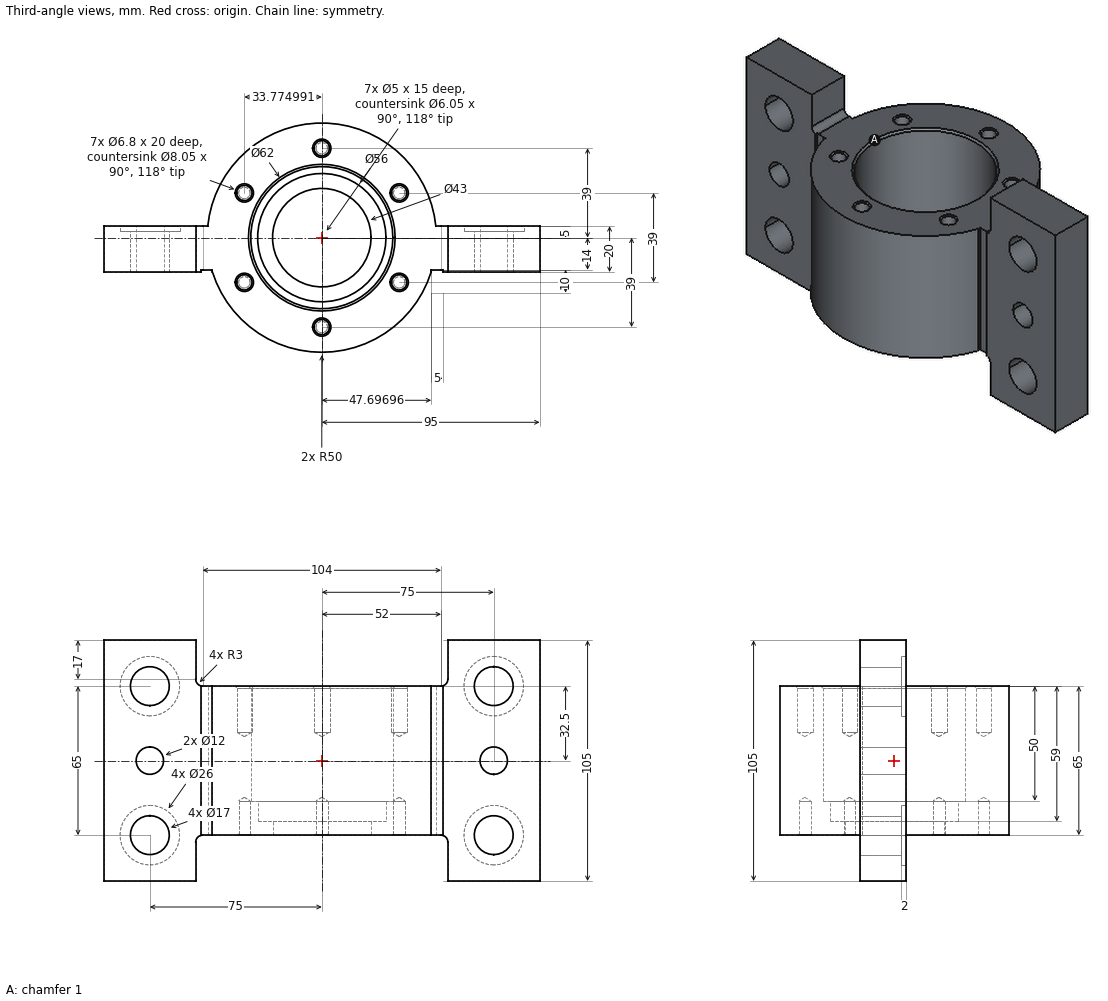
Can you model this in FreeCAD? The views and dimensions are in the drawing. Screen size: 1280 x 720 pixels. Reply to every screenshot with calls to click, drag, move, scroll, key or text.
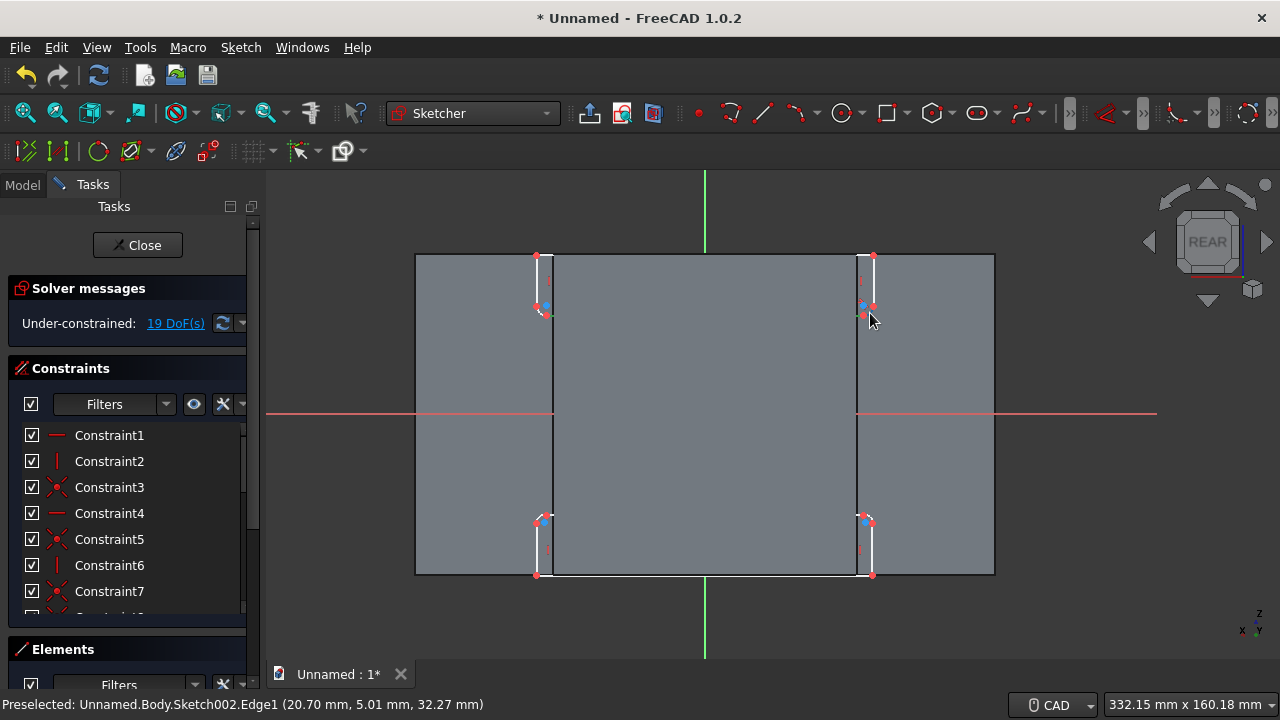
scroll(538, 311, up, 6)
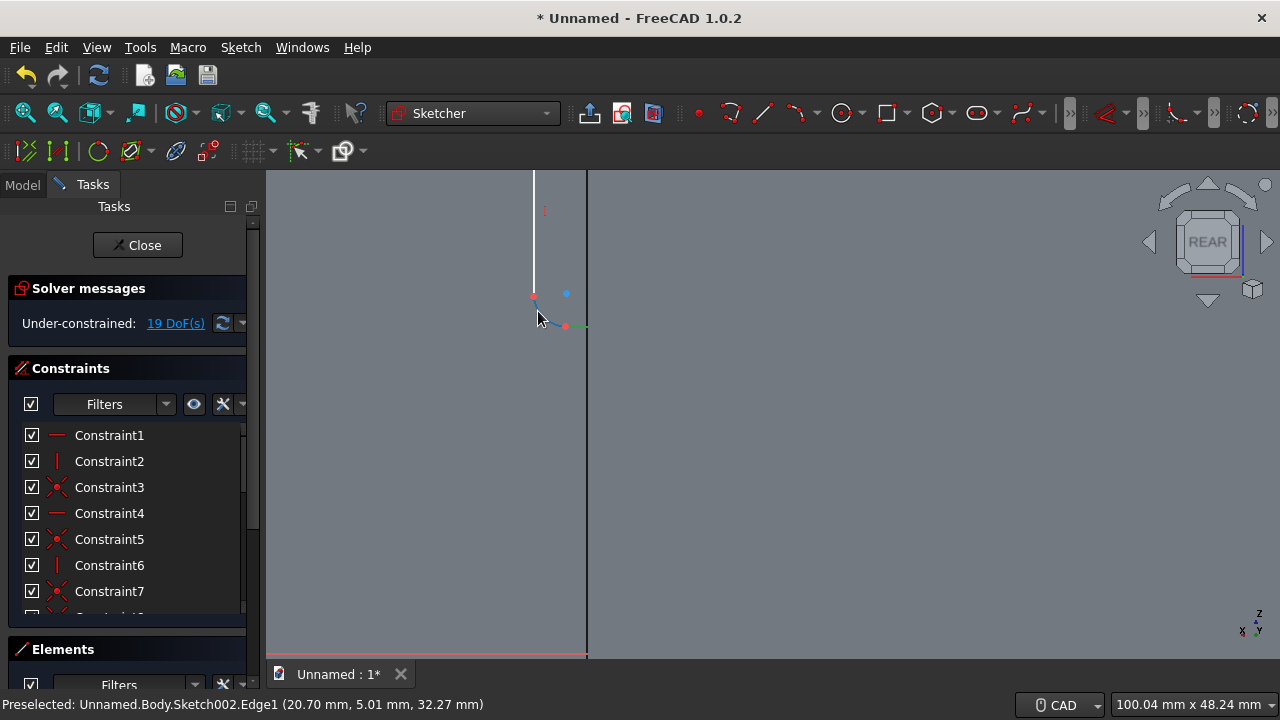
click(538, 310)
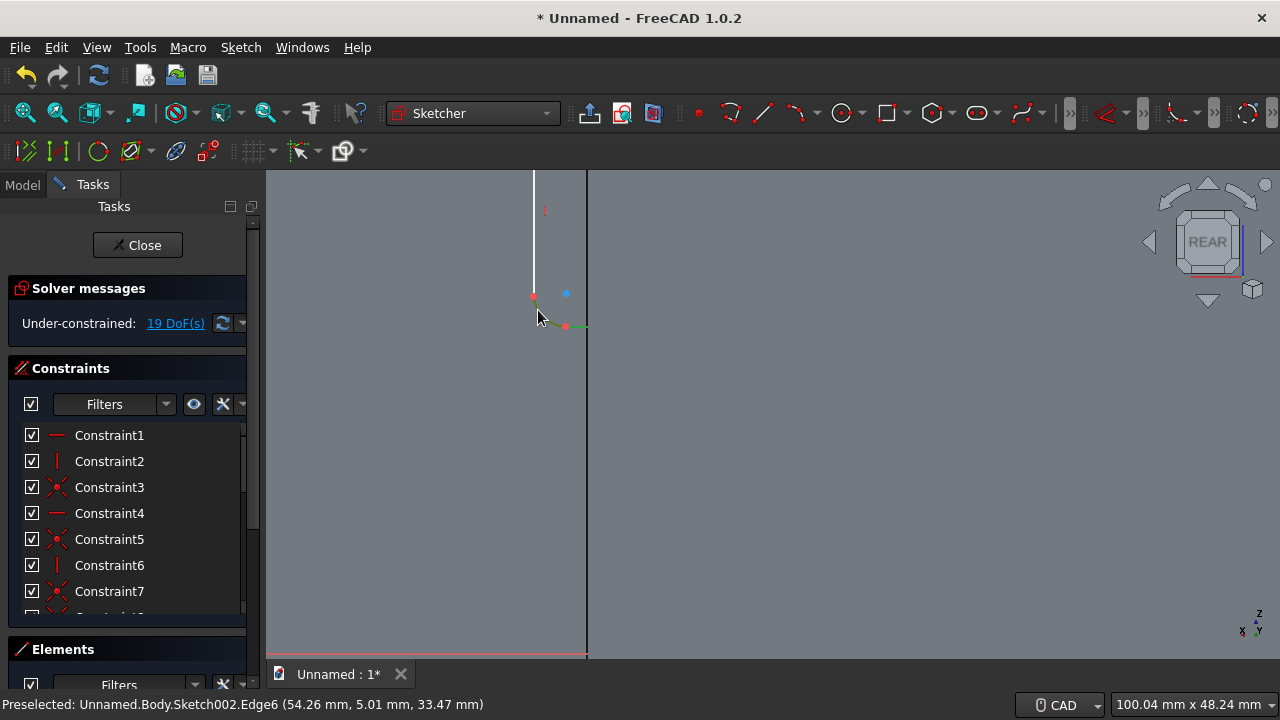
key(t)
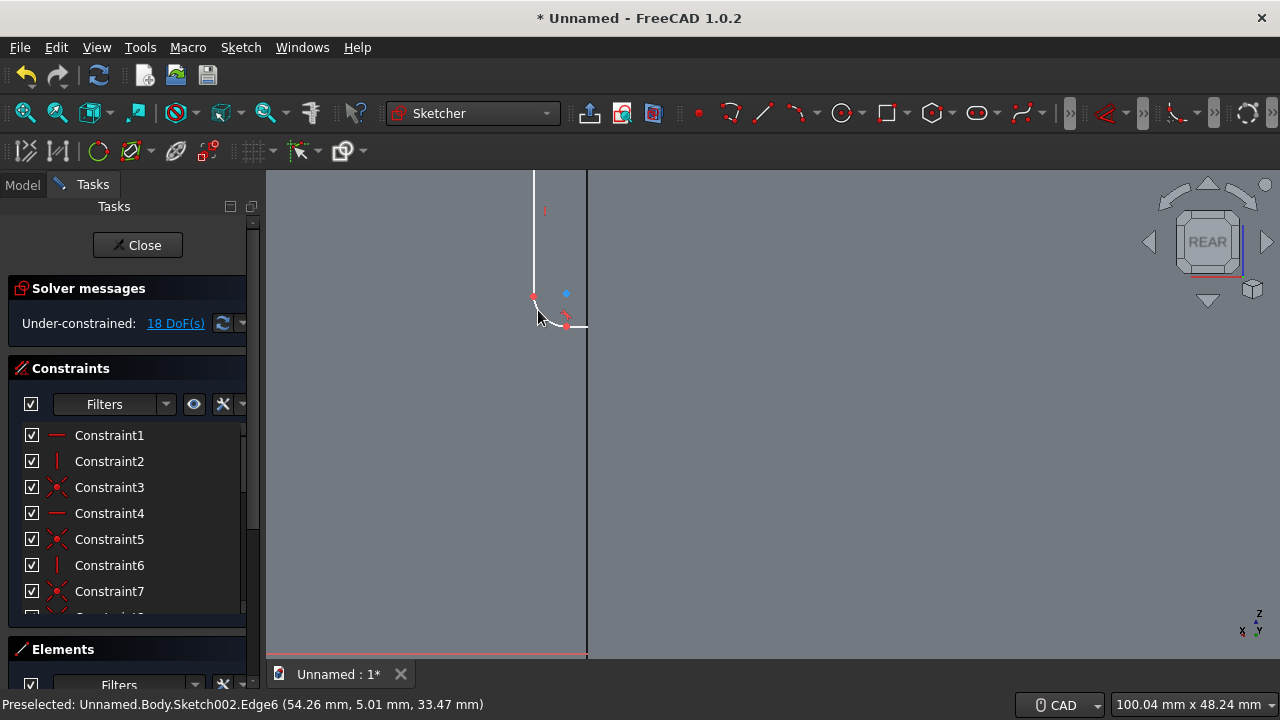
scroll(538, 311, down, 6)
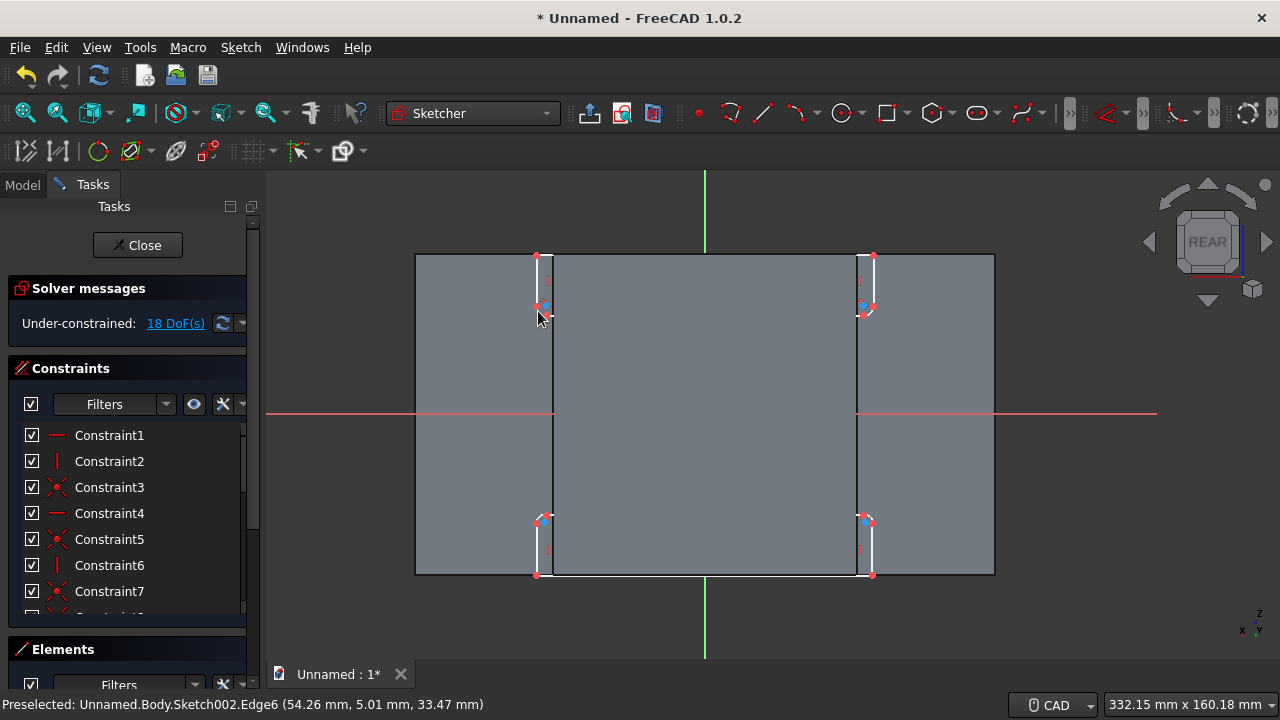
click(874, 291)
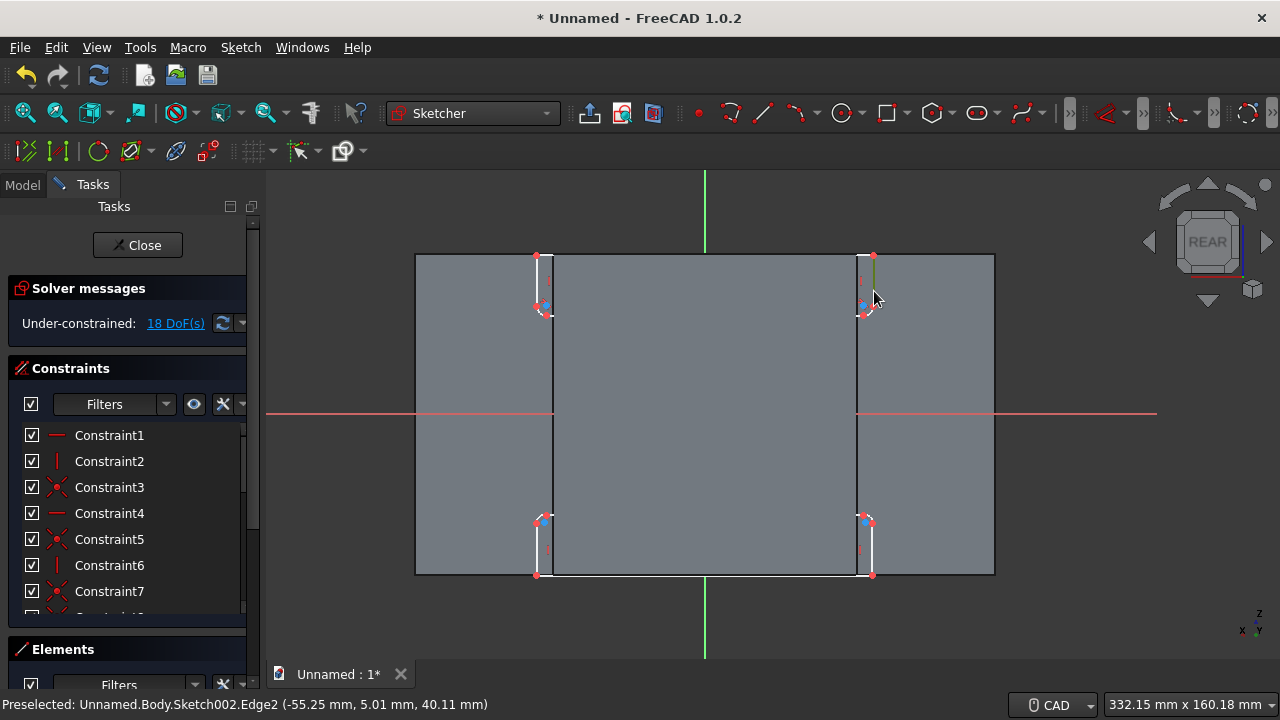
scroll(870, 313, up, 4)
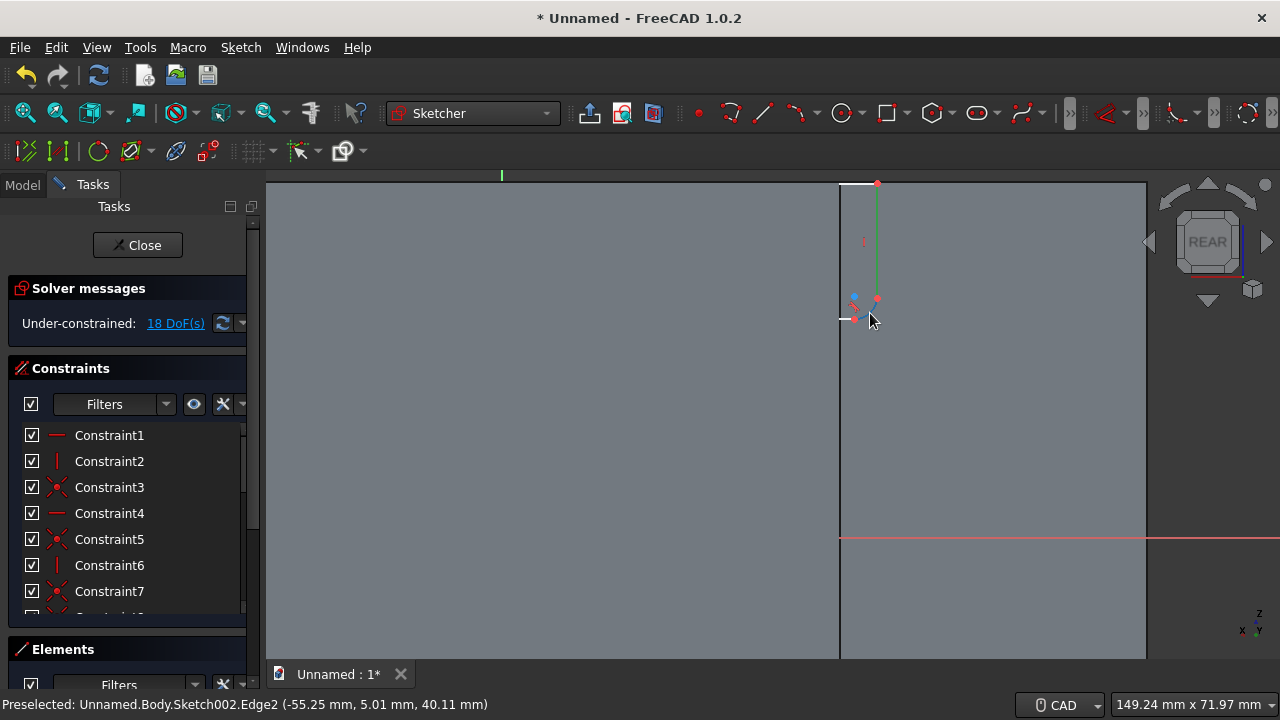
click(870, 313)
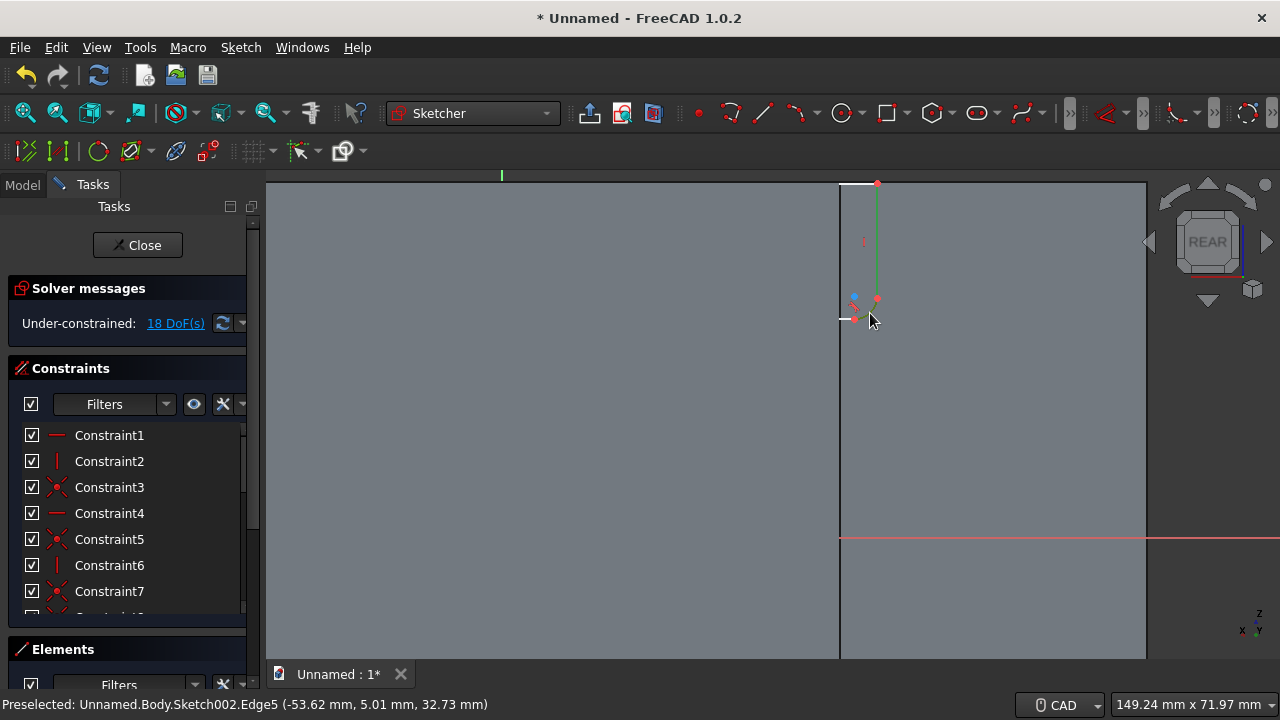
key(t)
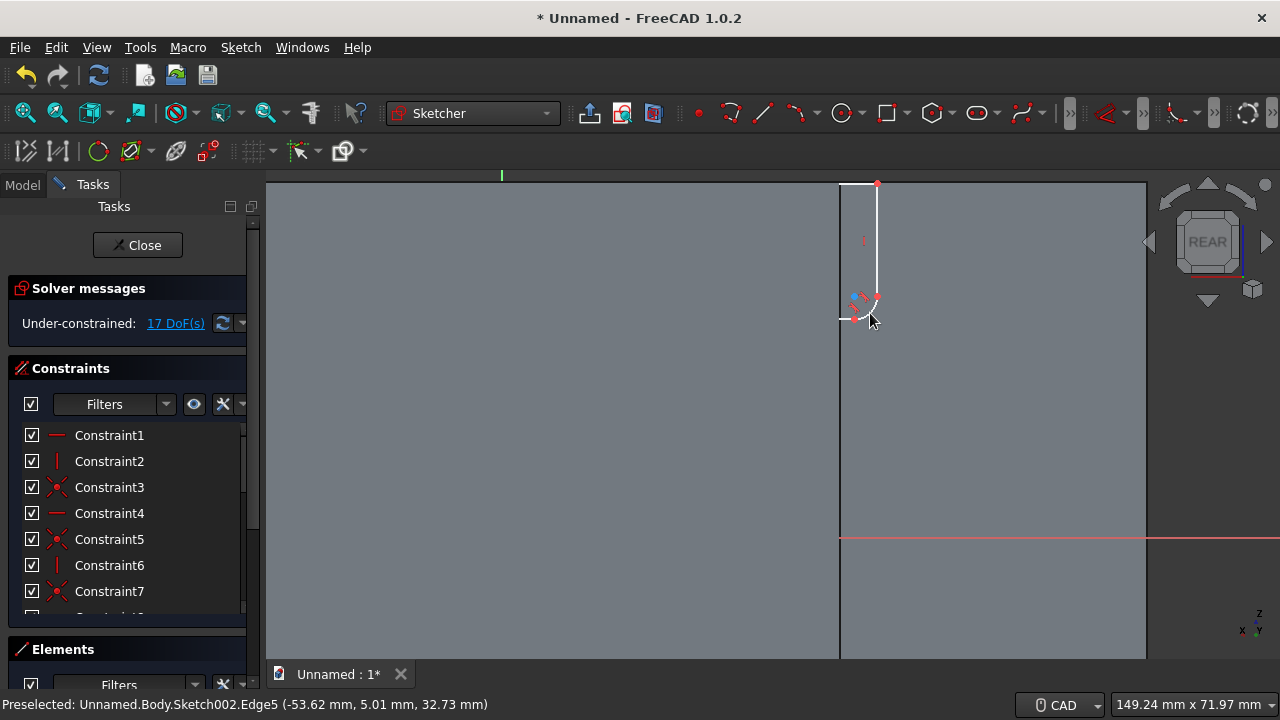
scroll(870, 313, down, 4)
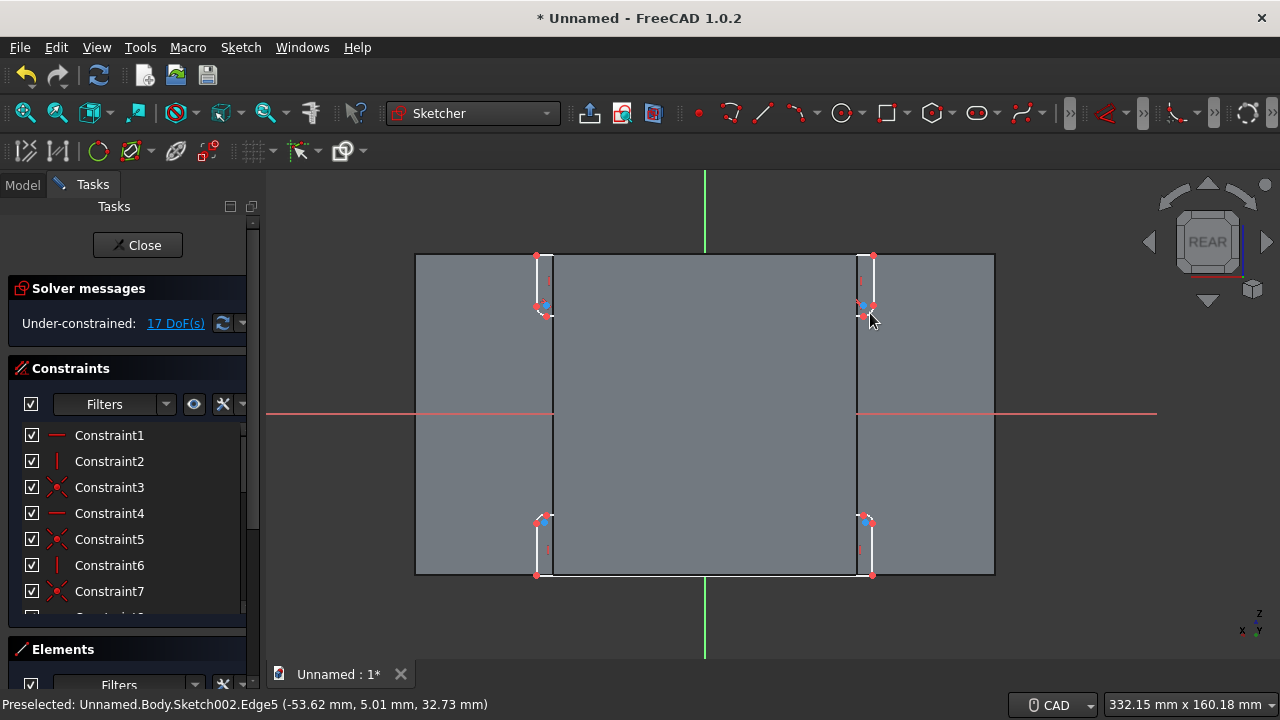
click(537, 271)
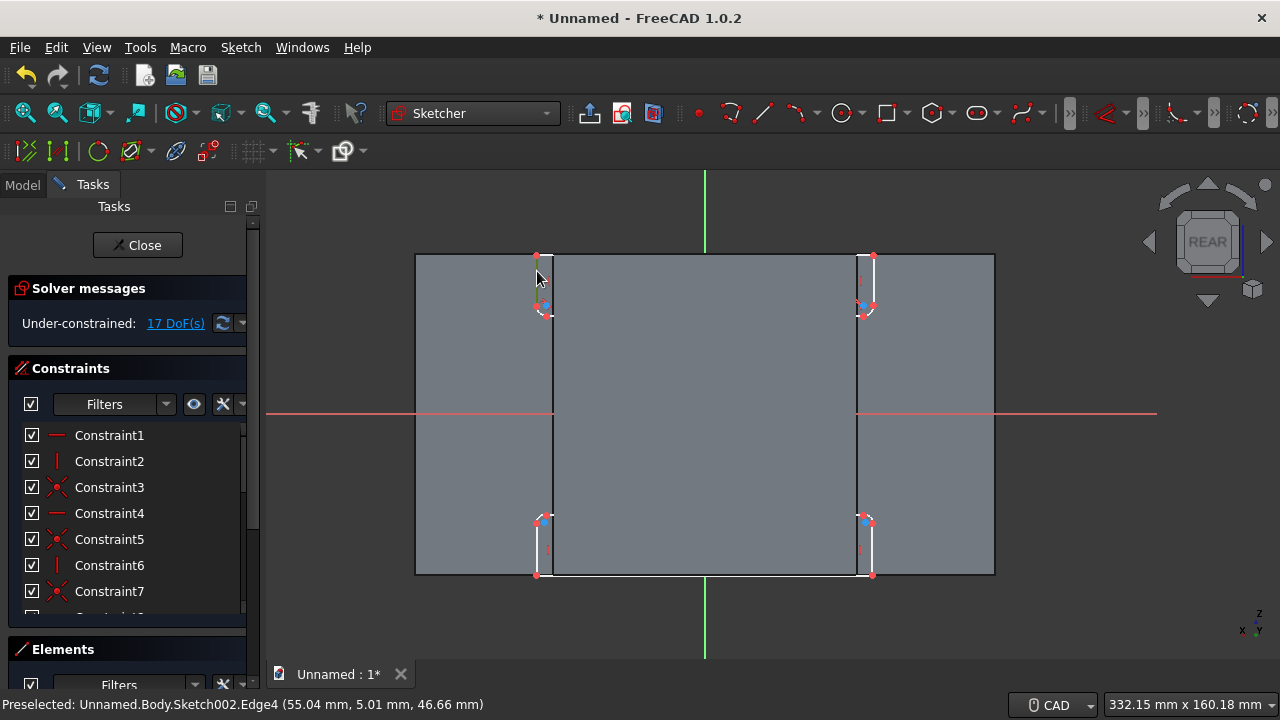
scroll(540, 313, up, 4)